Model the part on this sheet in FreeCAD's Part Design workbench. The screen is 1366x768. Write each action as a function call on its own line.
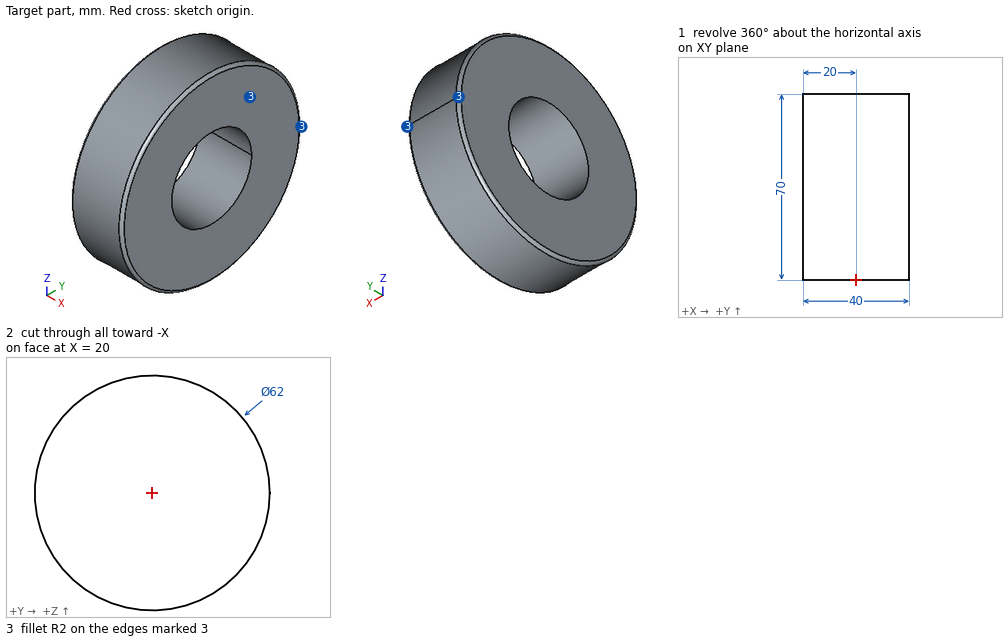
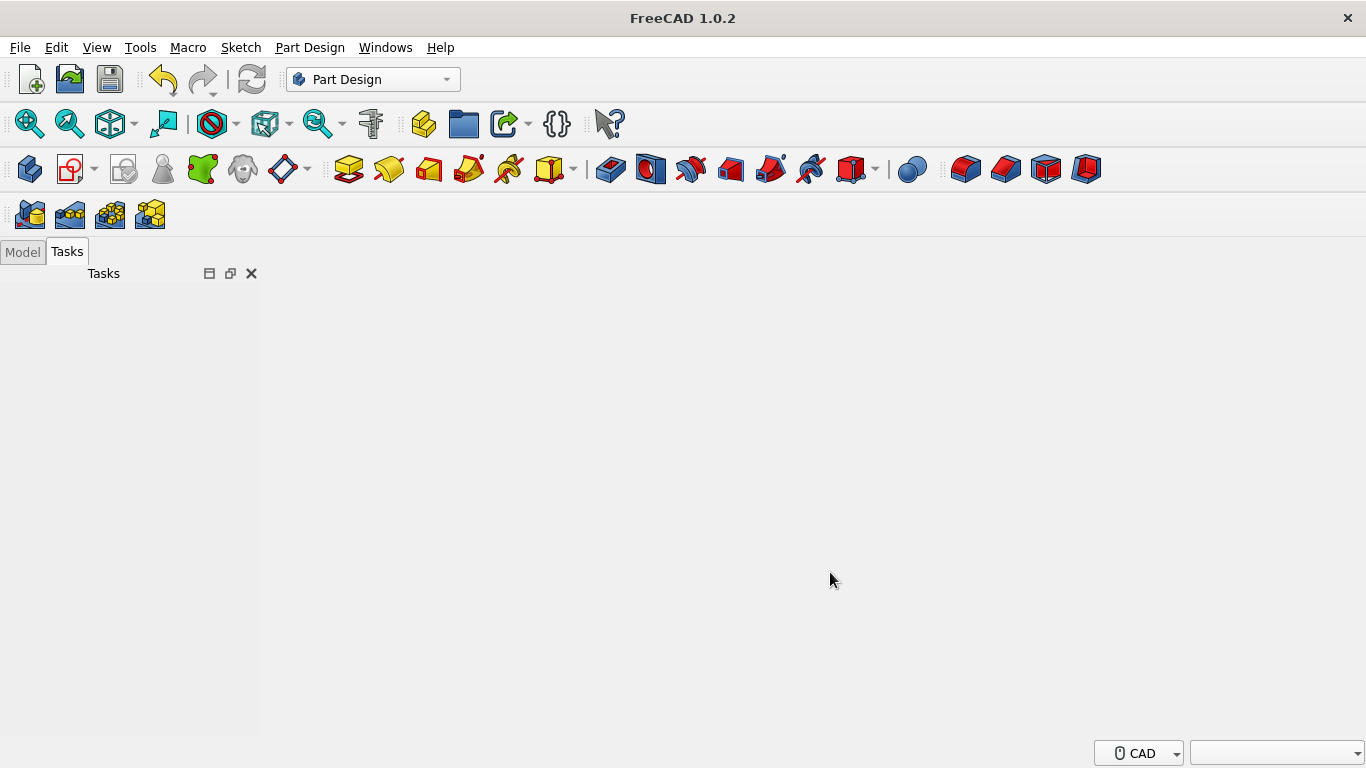
key(ctrl+n)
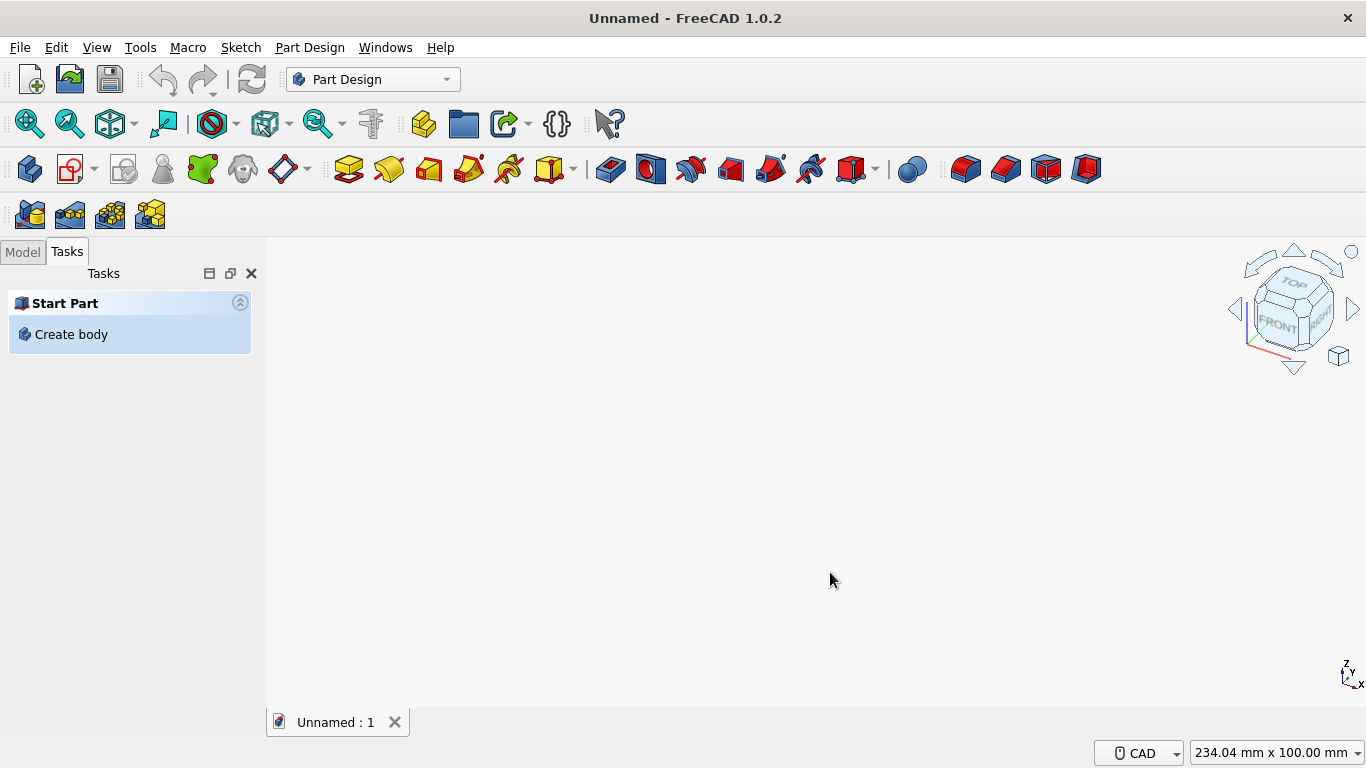
click(70, 170)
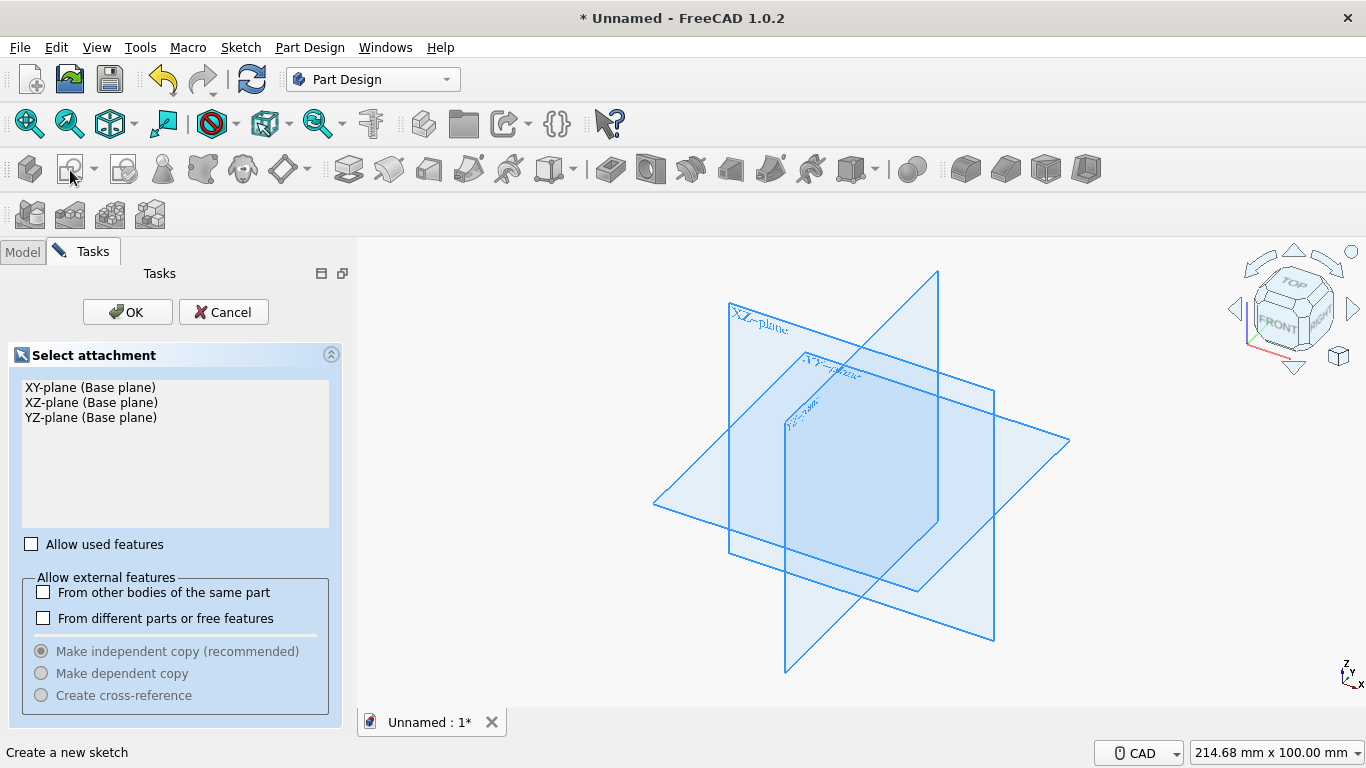
click(82, 388)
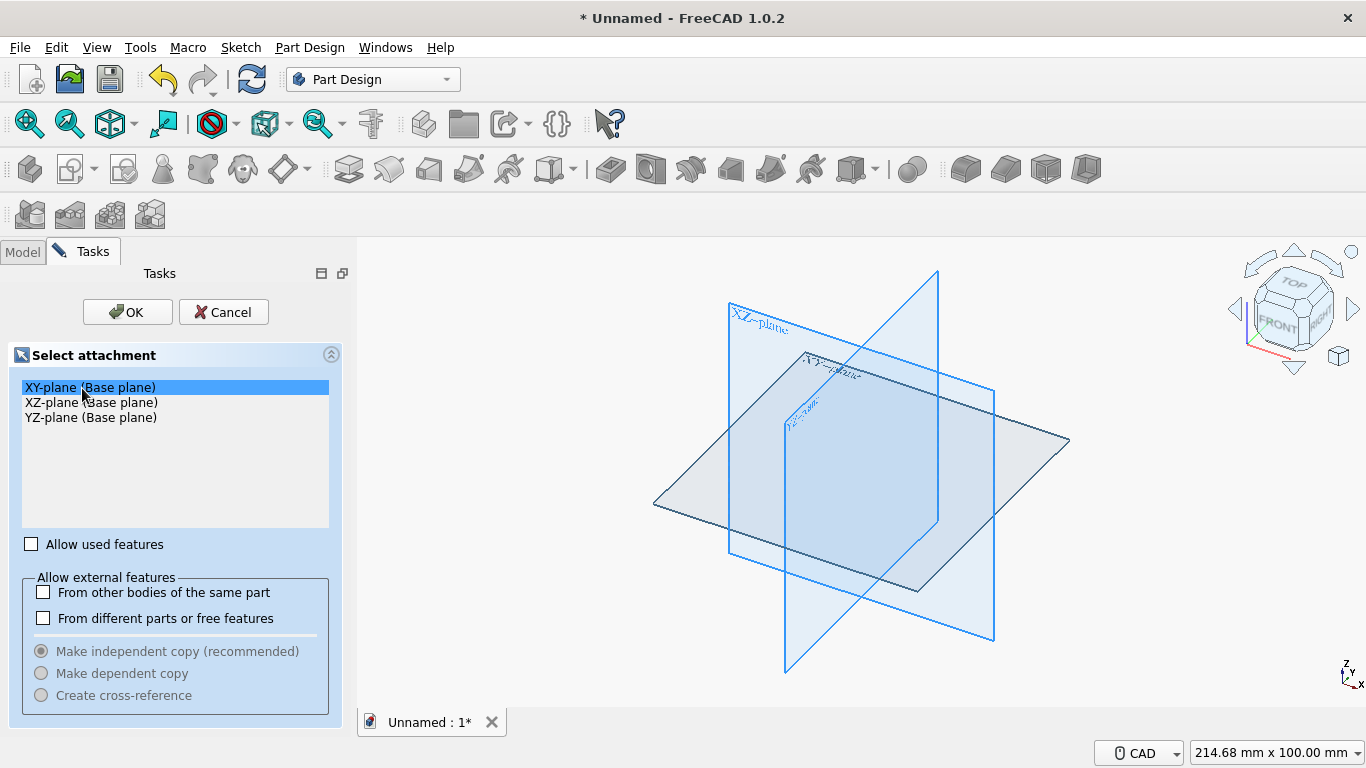
click(128, 312)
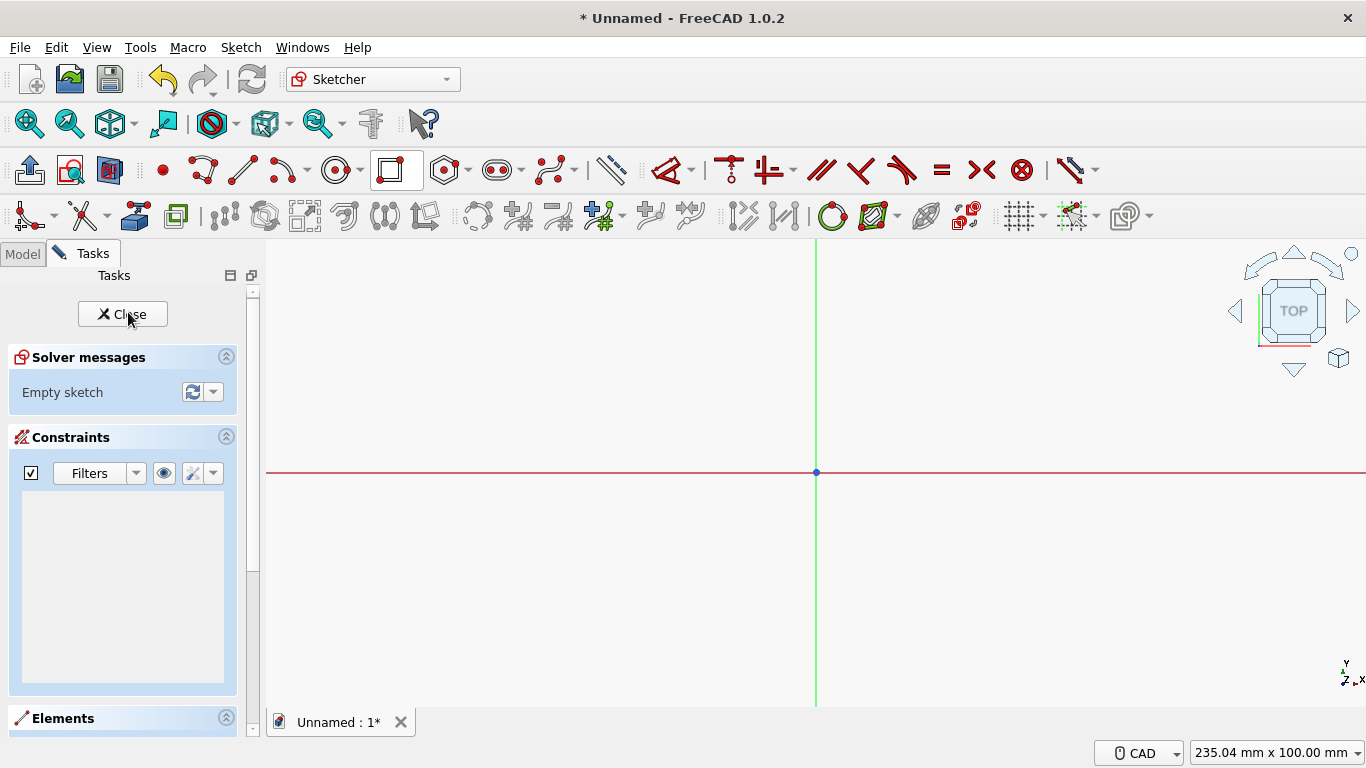
scroll(608, 679, down, 2)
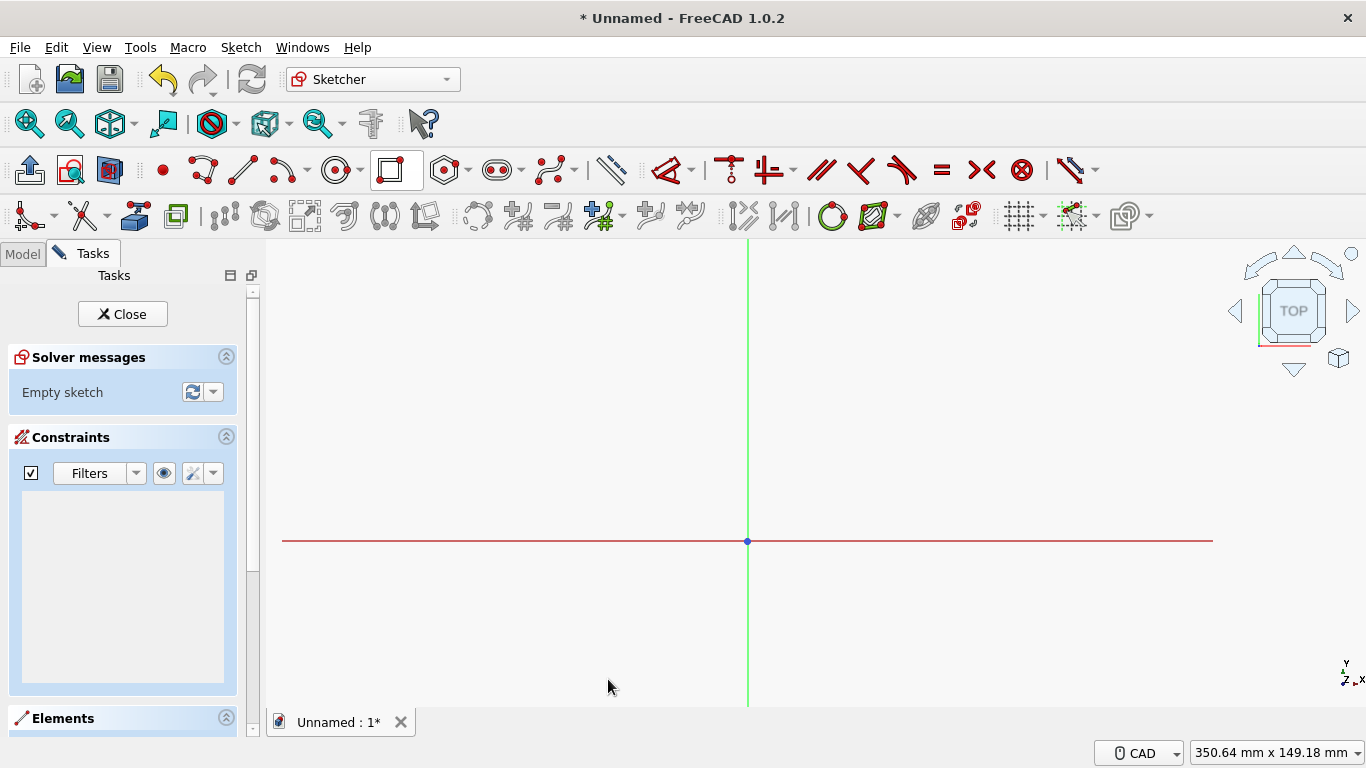
key(g)
key(r)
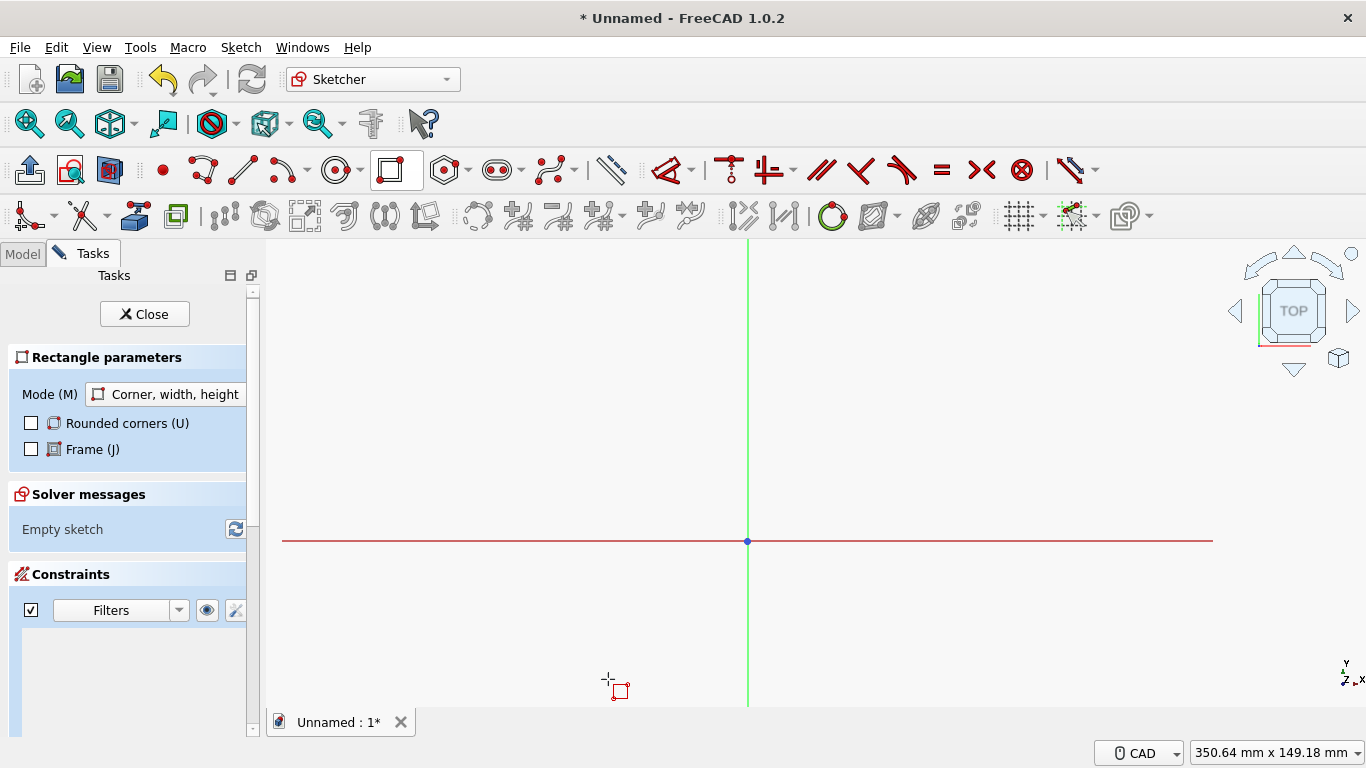
click(685, 322)
click(810, 541)
key(Escape)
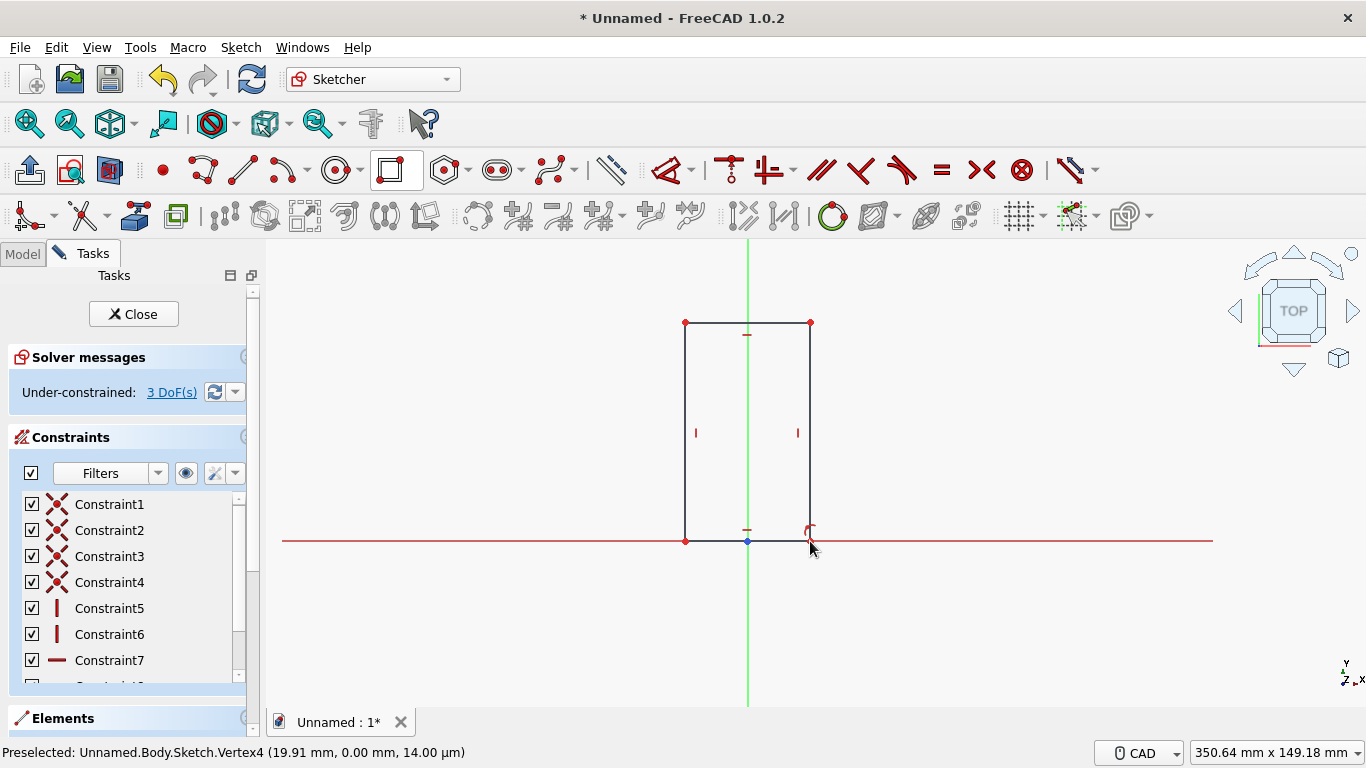
click(685, 388)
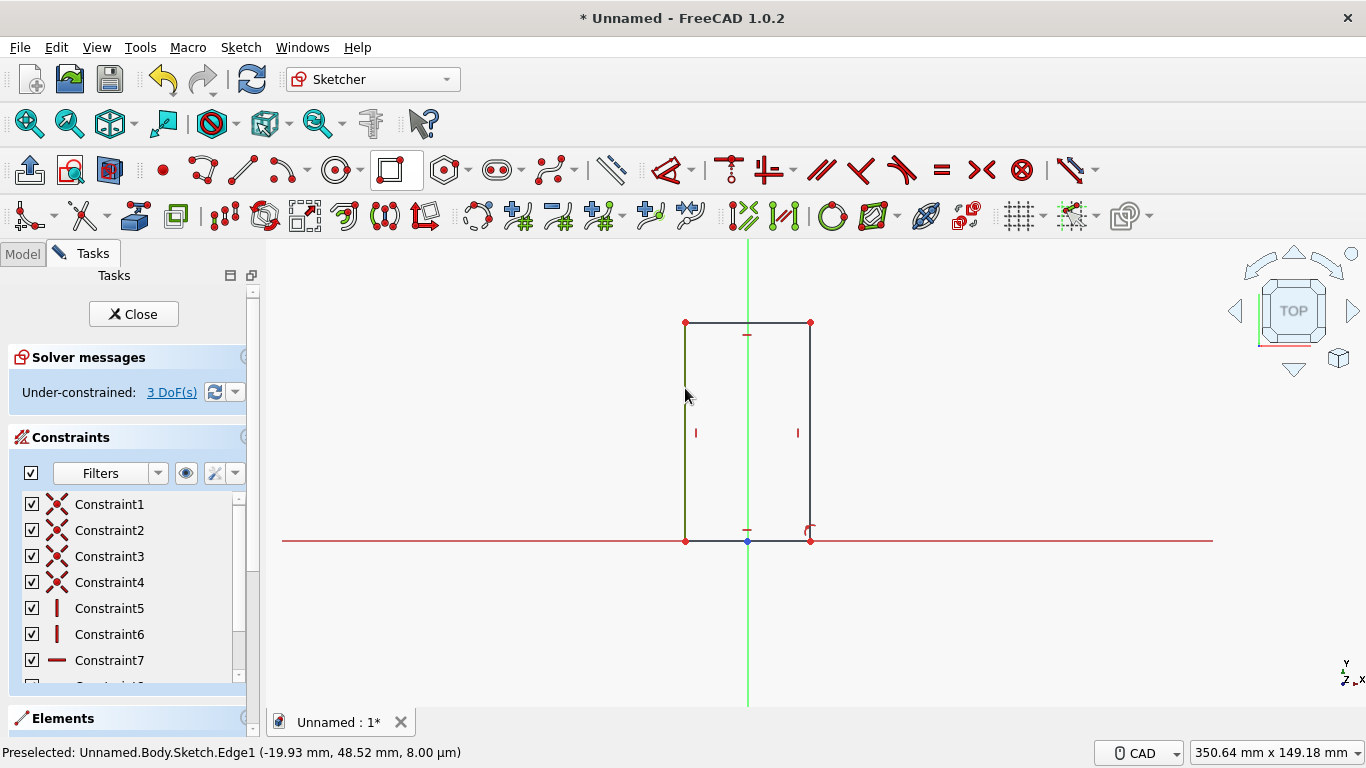
key(i)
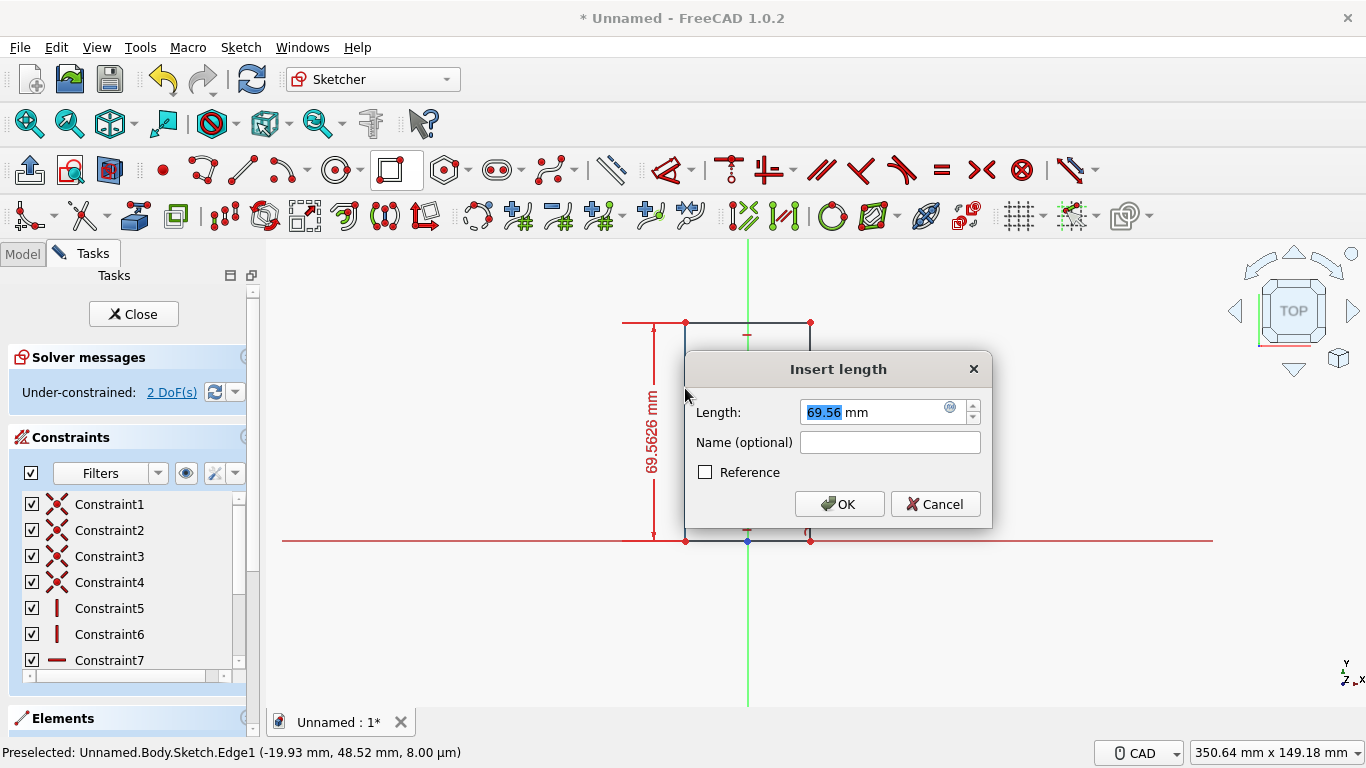
text(70)
key(Return)